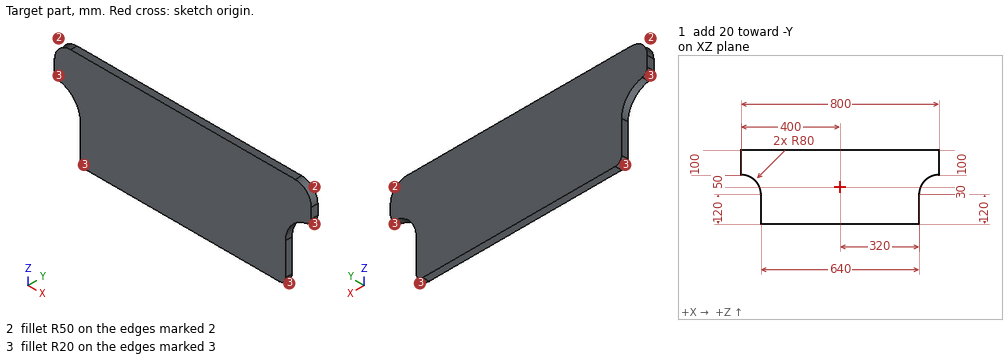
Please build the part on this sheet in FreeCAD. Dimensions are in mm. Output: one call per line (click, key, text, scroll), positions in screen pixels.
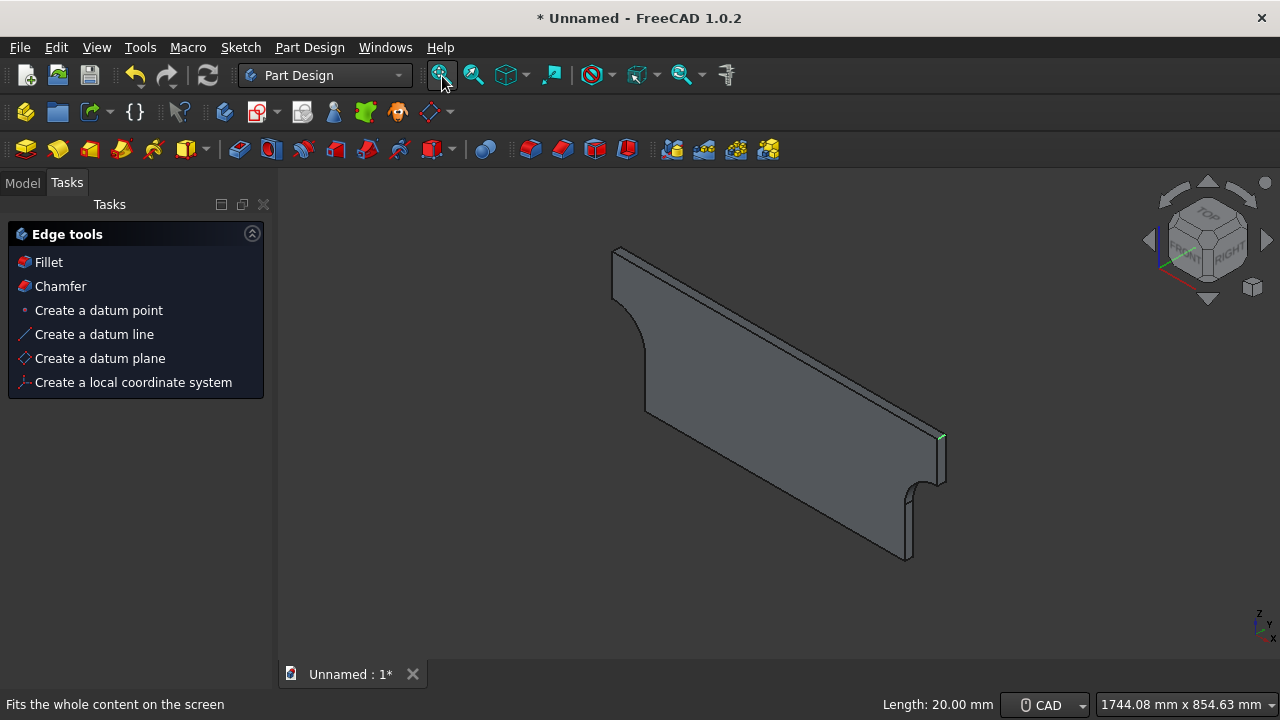
scroll(617, 248, up, 7)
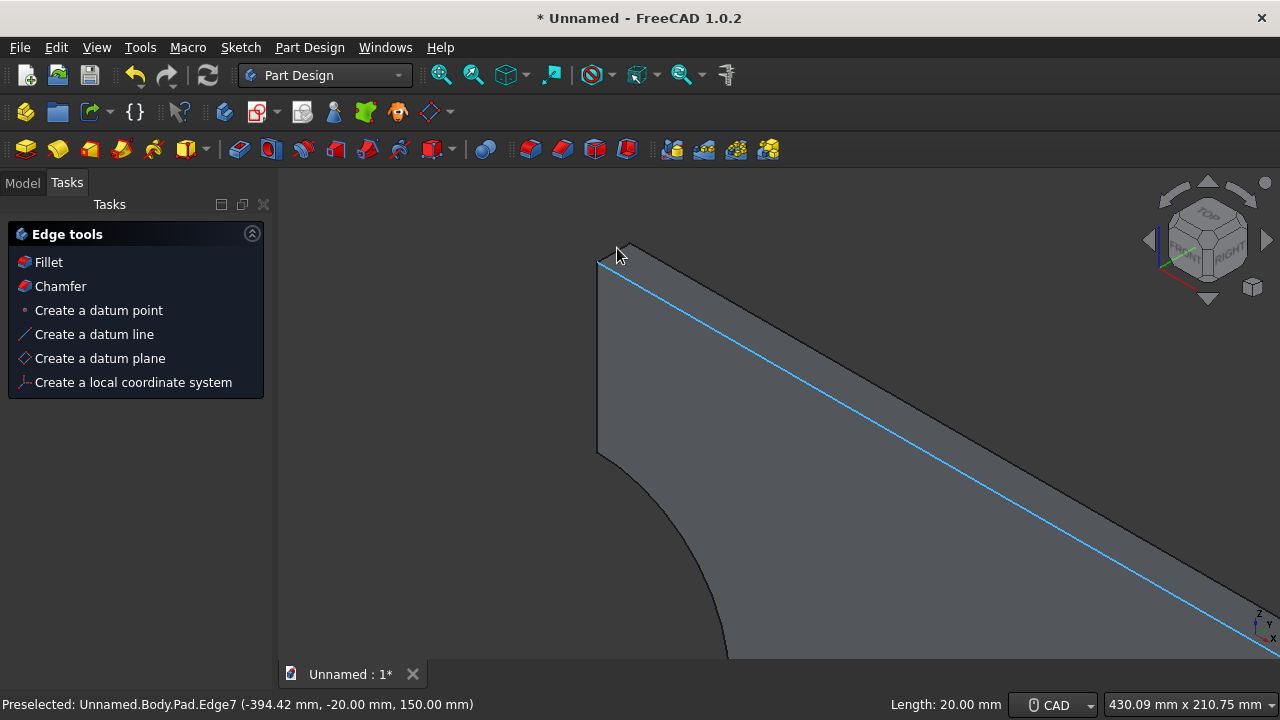
key(v)
key(f)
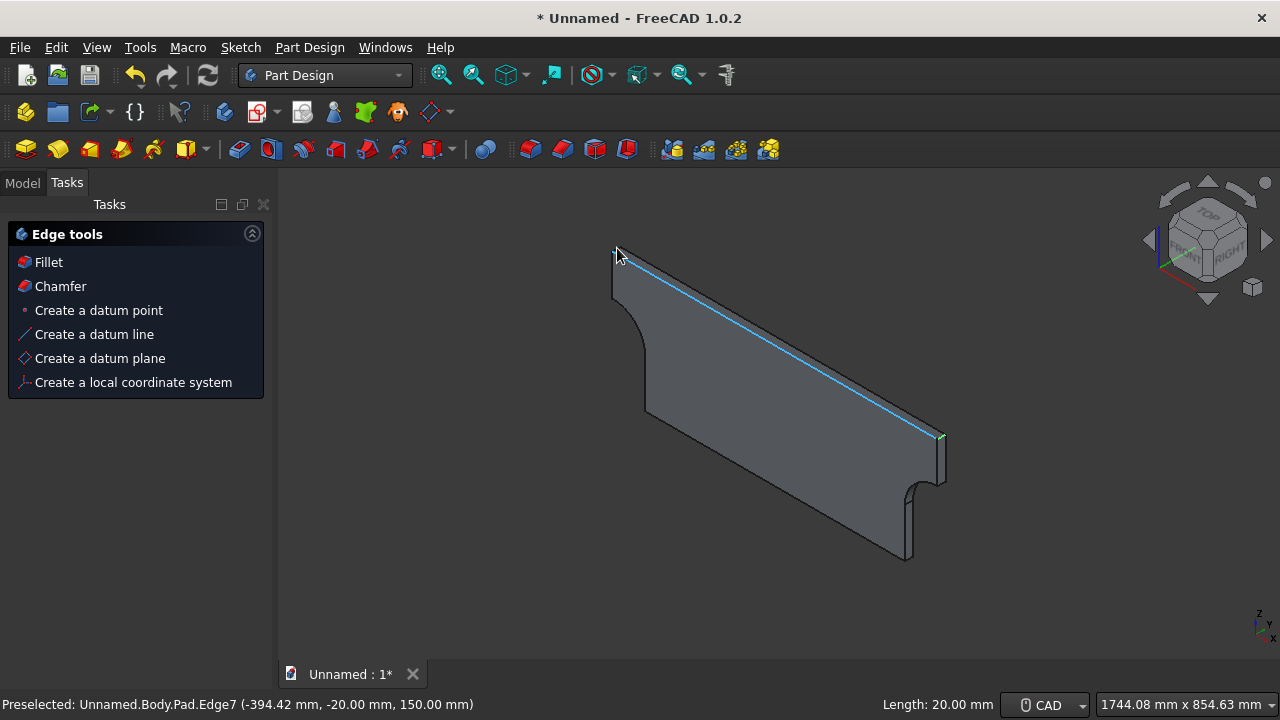
key(2)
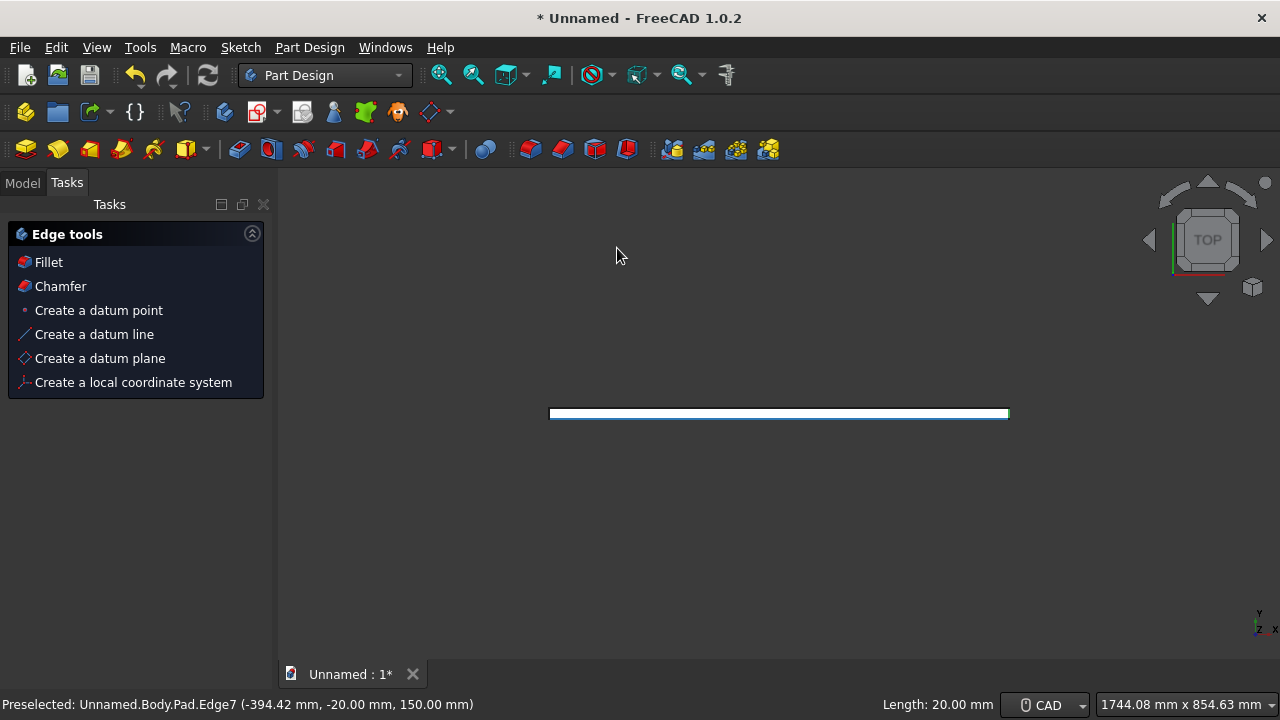
click(549, 414, ctrl)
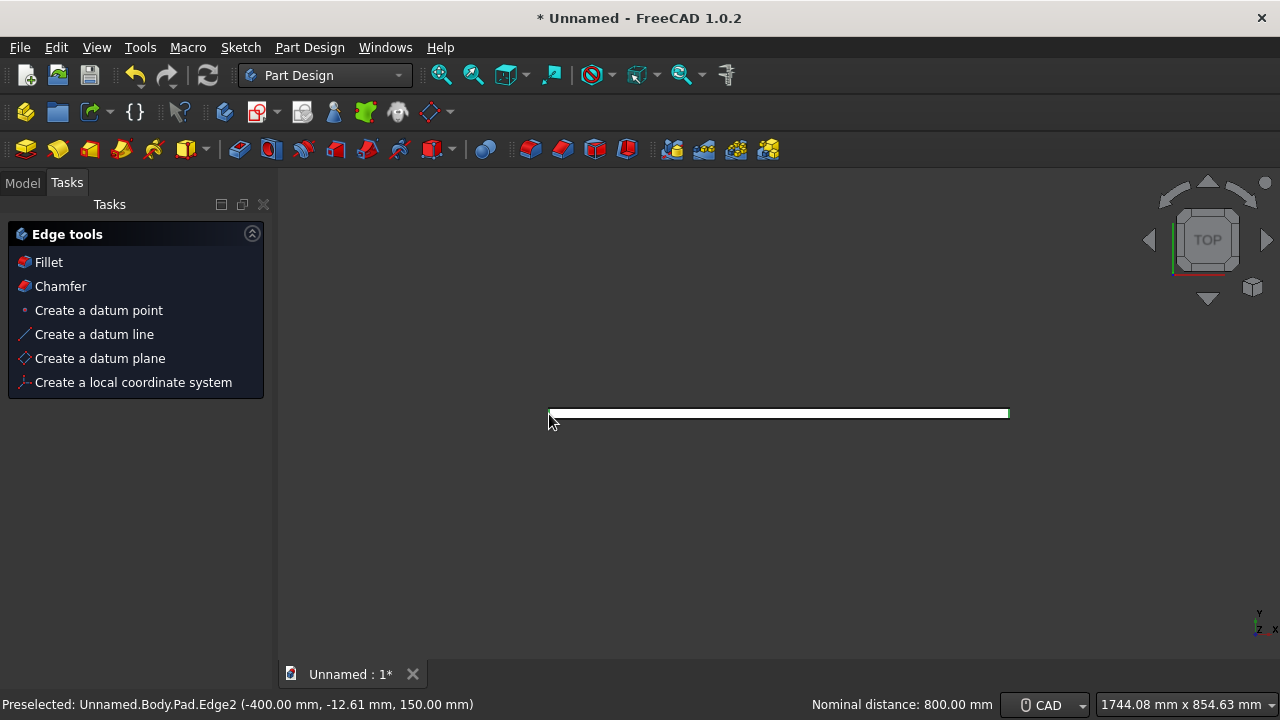
click(532, 150)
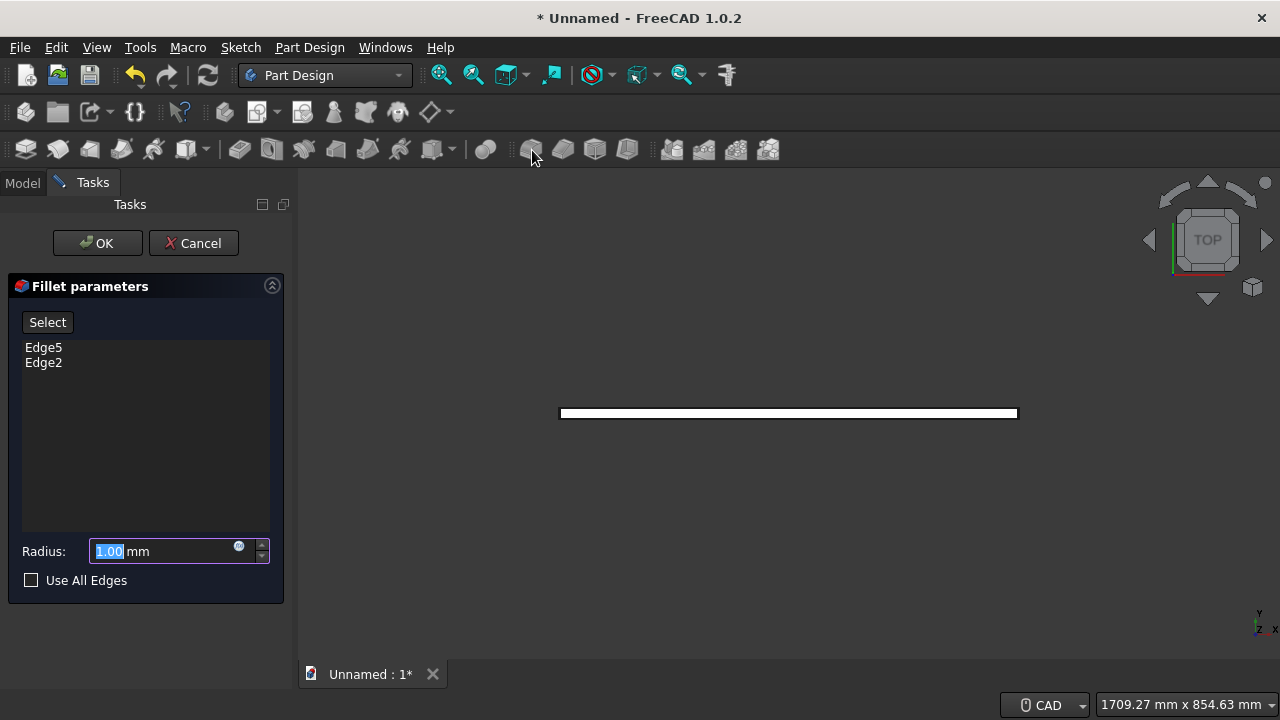
text(50)
key(Tab)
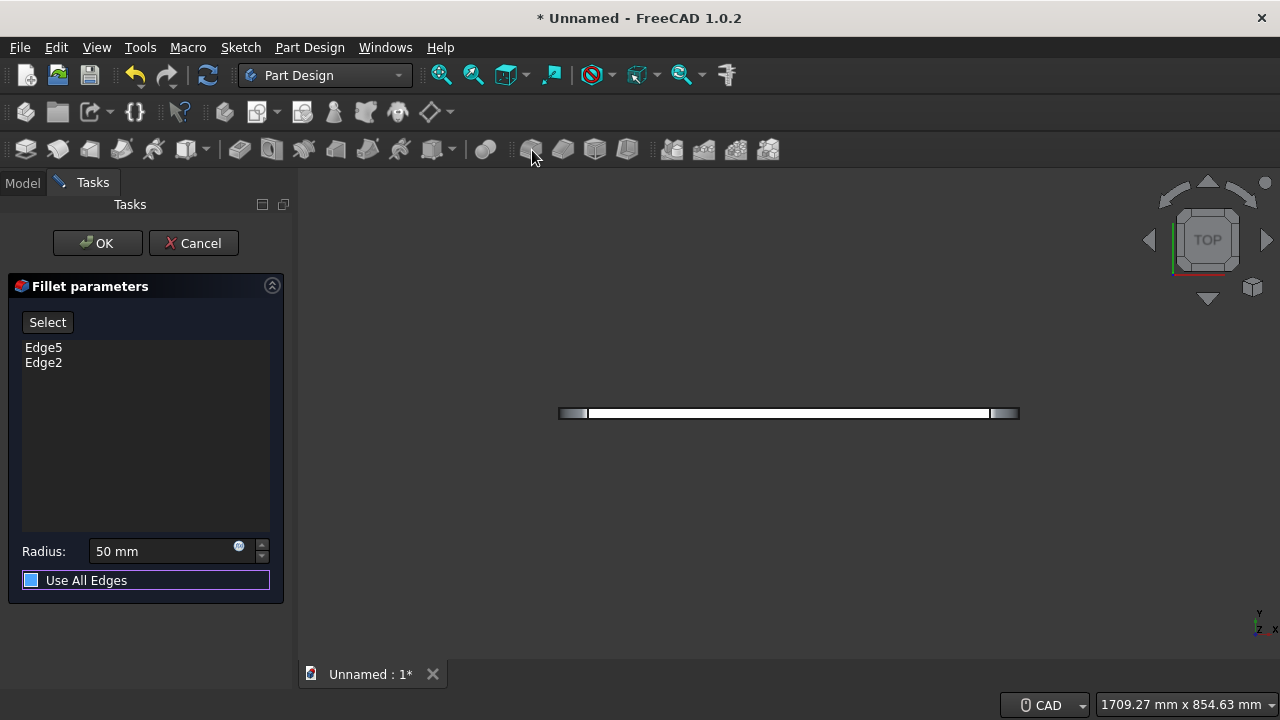
click(98, 243)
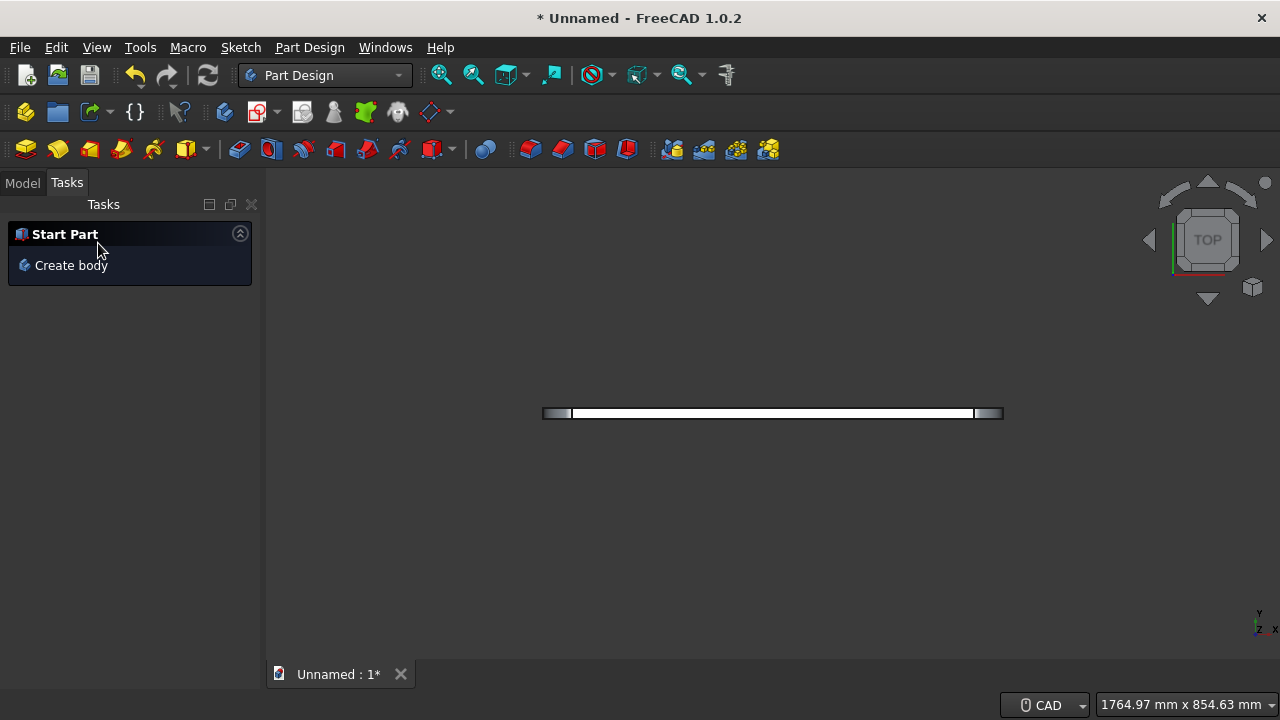
scroll(543, 412, up, 7)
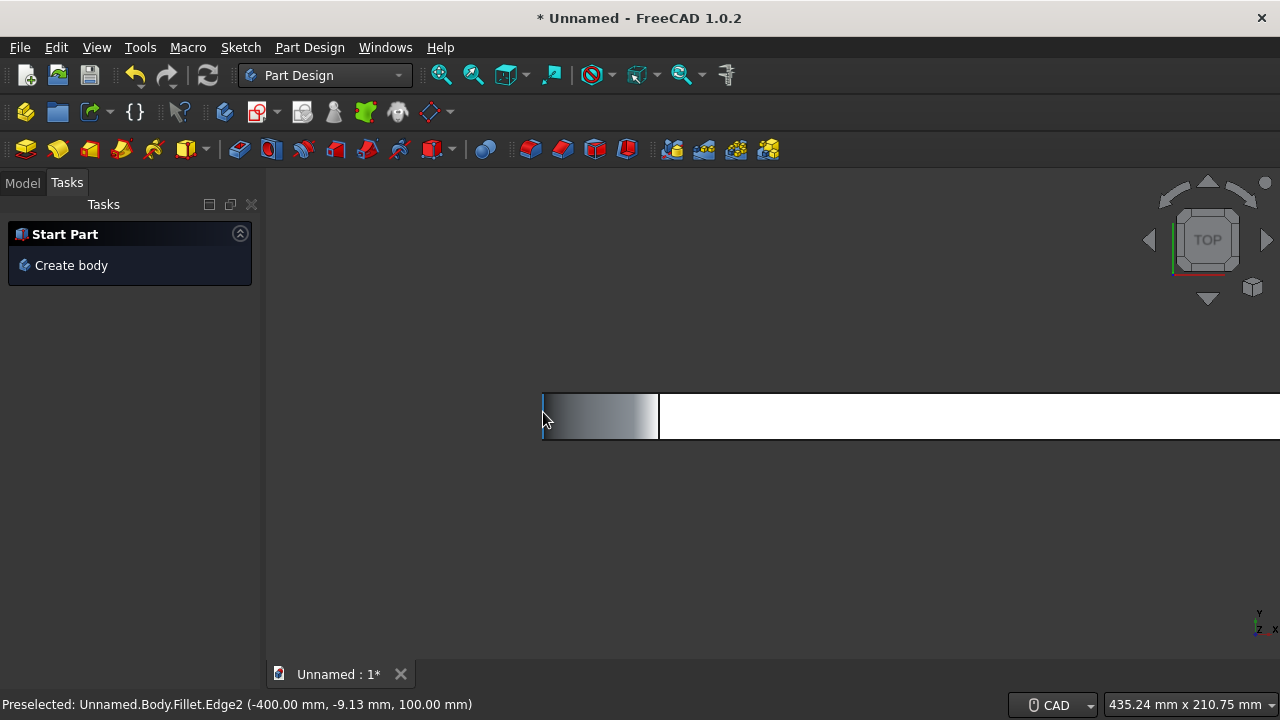
click(442, 76)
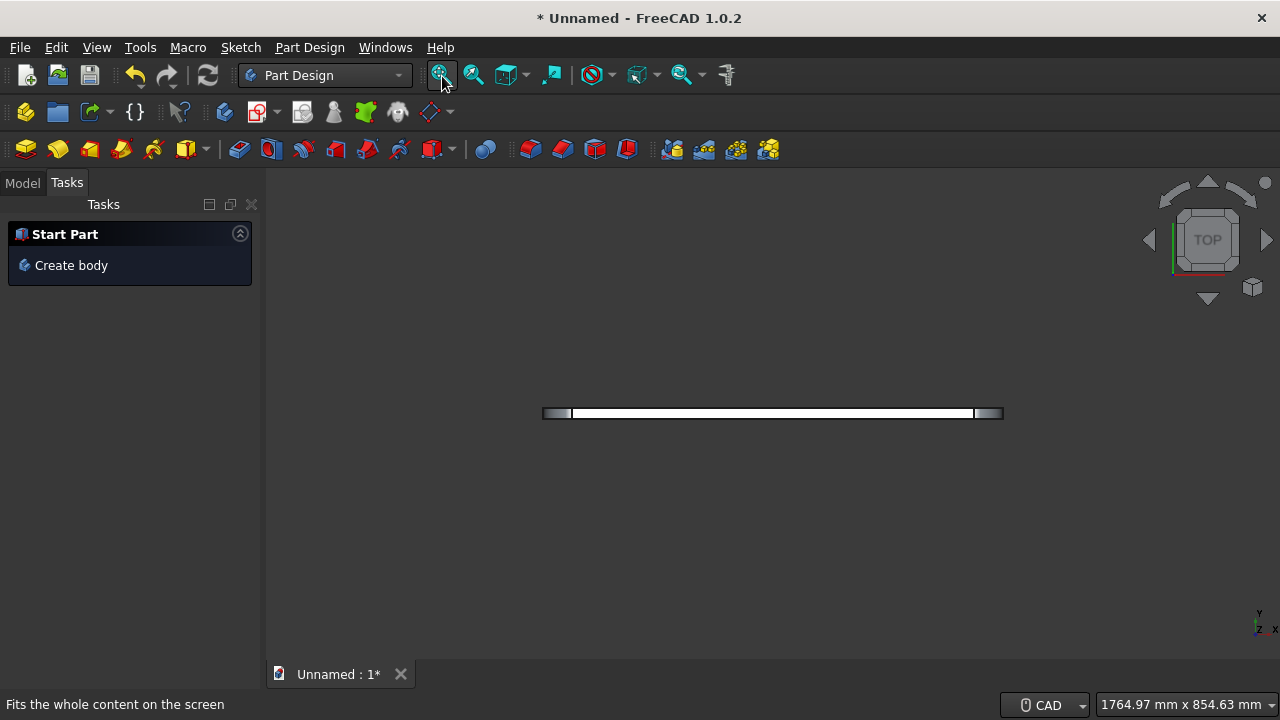
key(0)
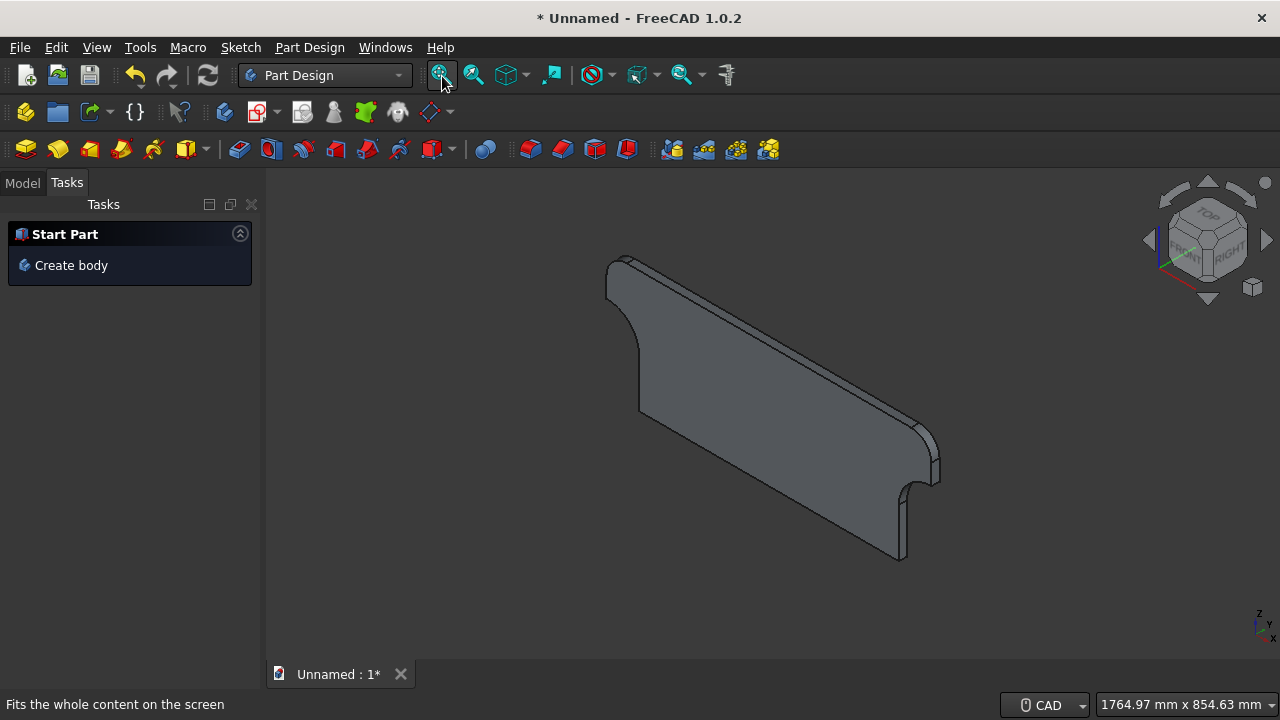
scroll(611, 295, up, 7)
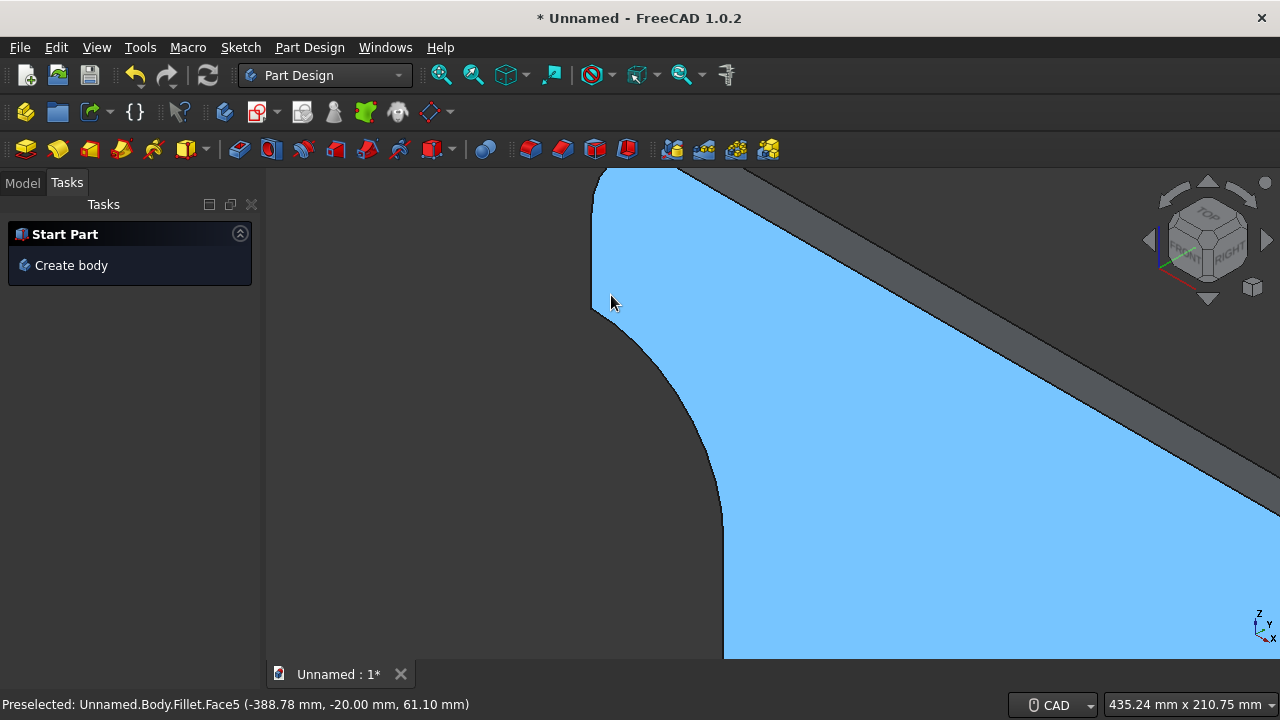
key(v)
key(f)